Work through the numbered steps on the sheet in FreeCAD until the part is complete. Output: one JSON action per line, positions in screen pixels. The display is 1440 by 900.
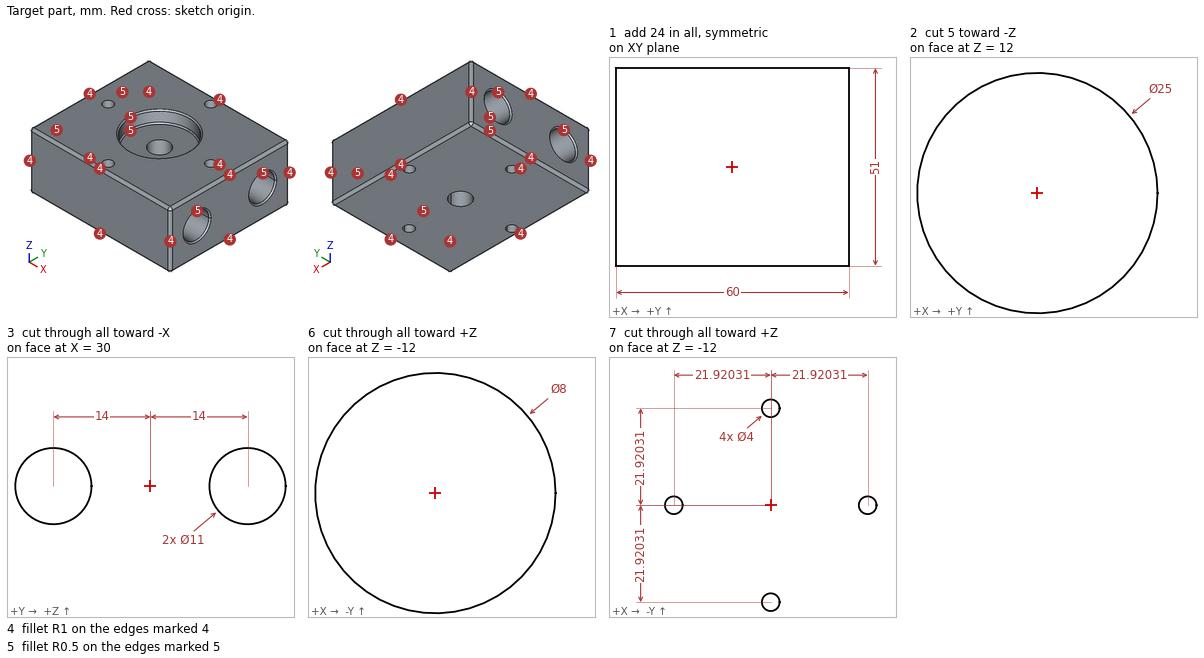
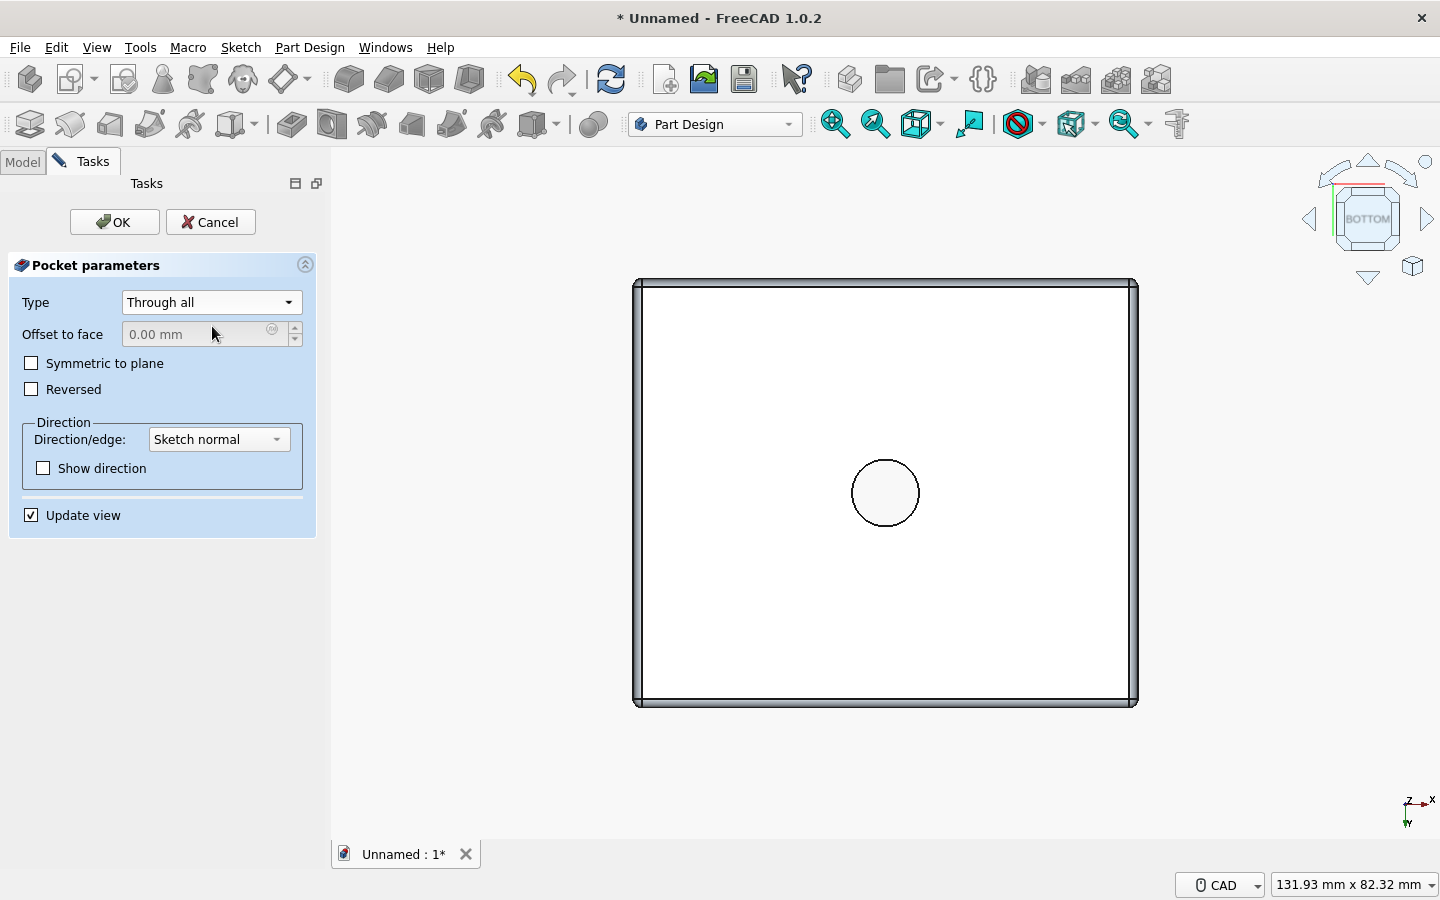
{"action": "left_click", "coordinate": [115, 222]}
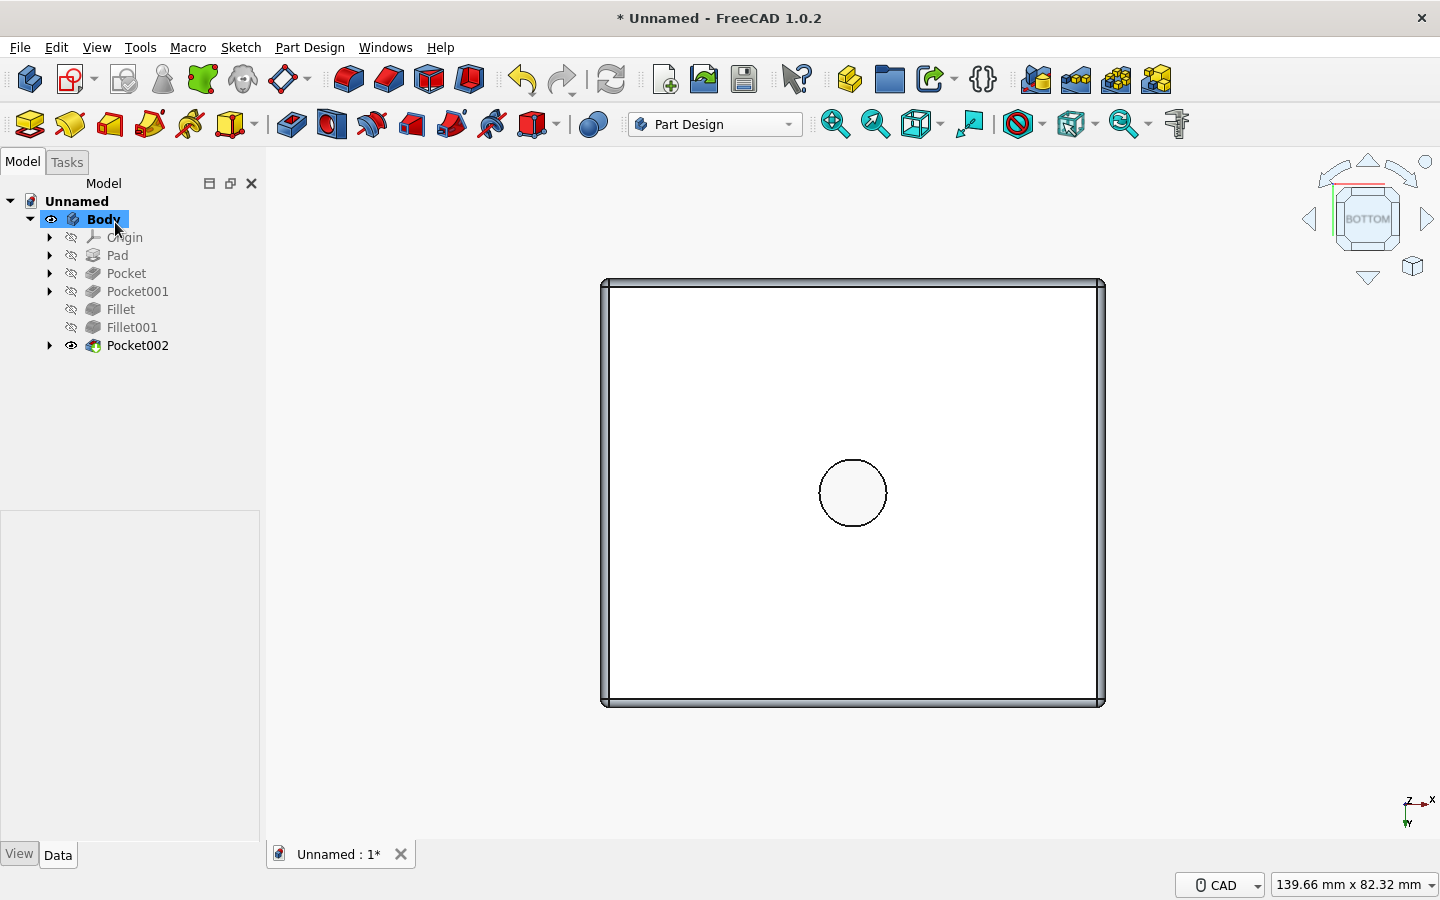
{"action": "left_click", "coordinate": [992, 551]}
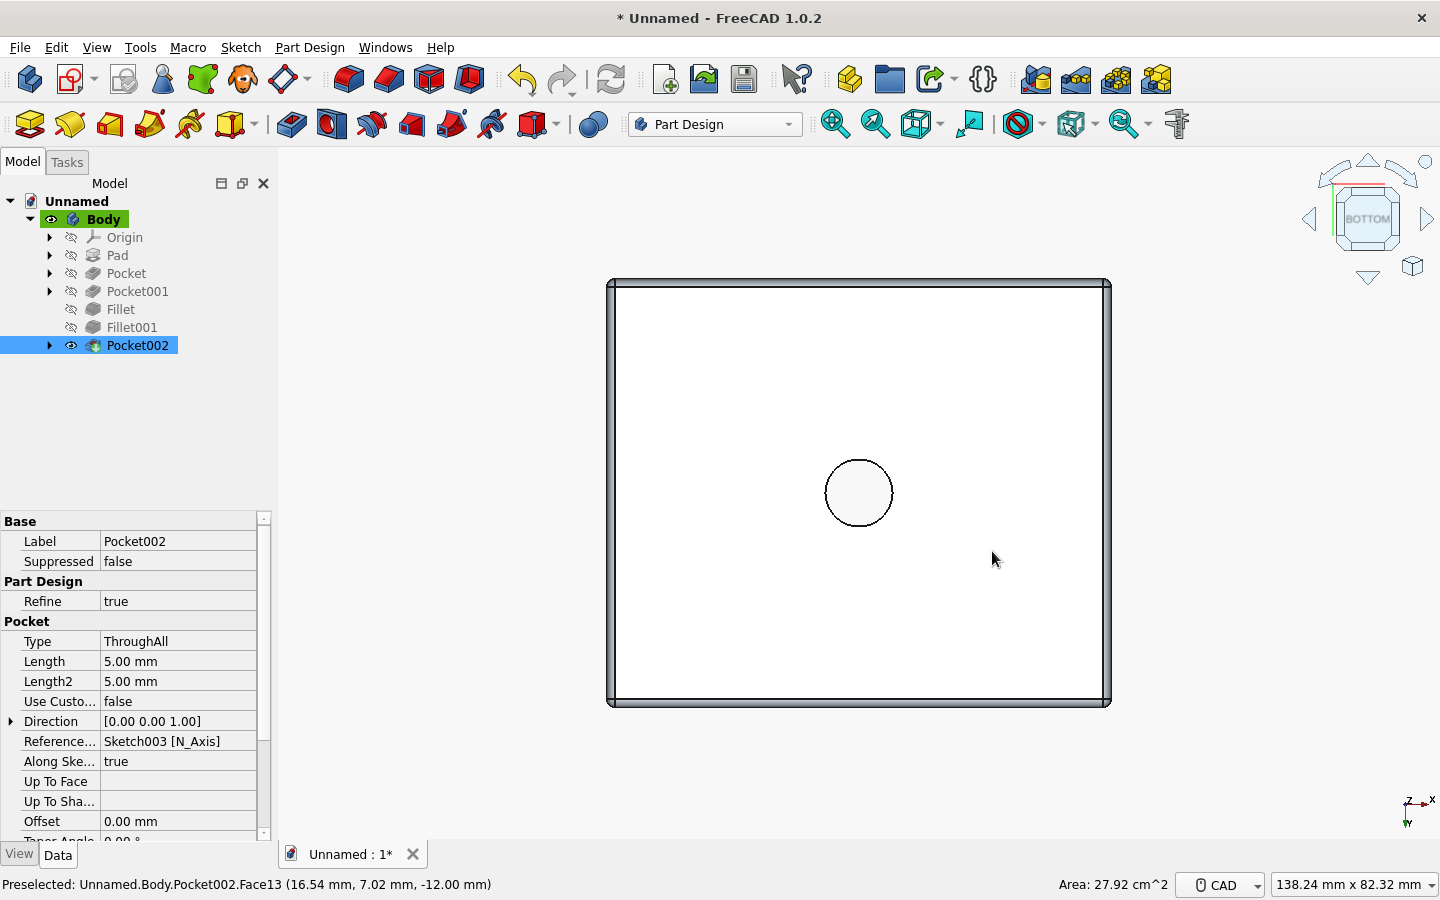
{"action": "left_click", "coordinate": [70, 80]}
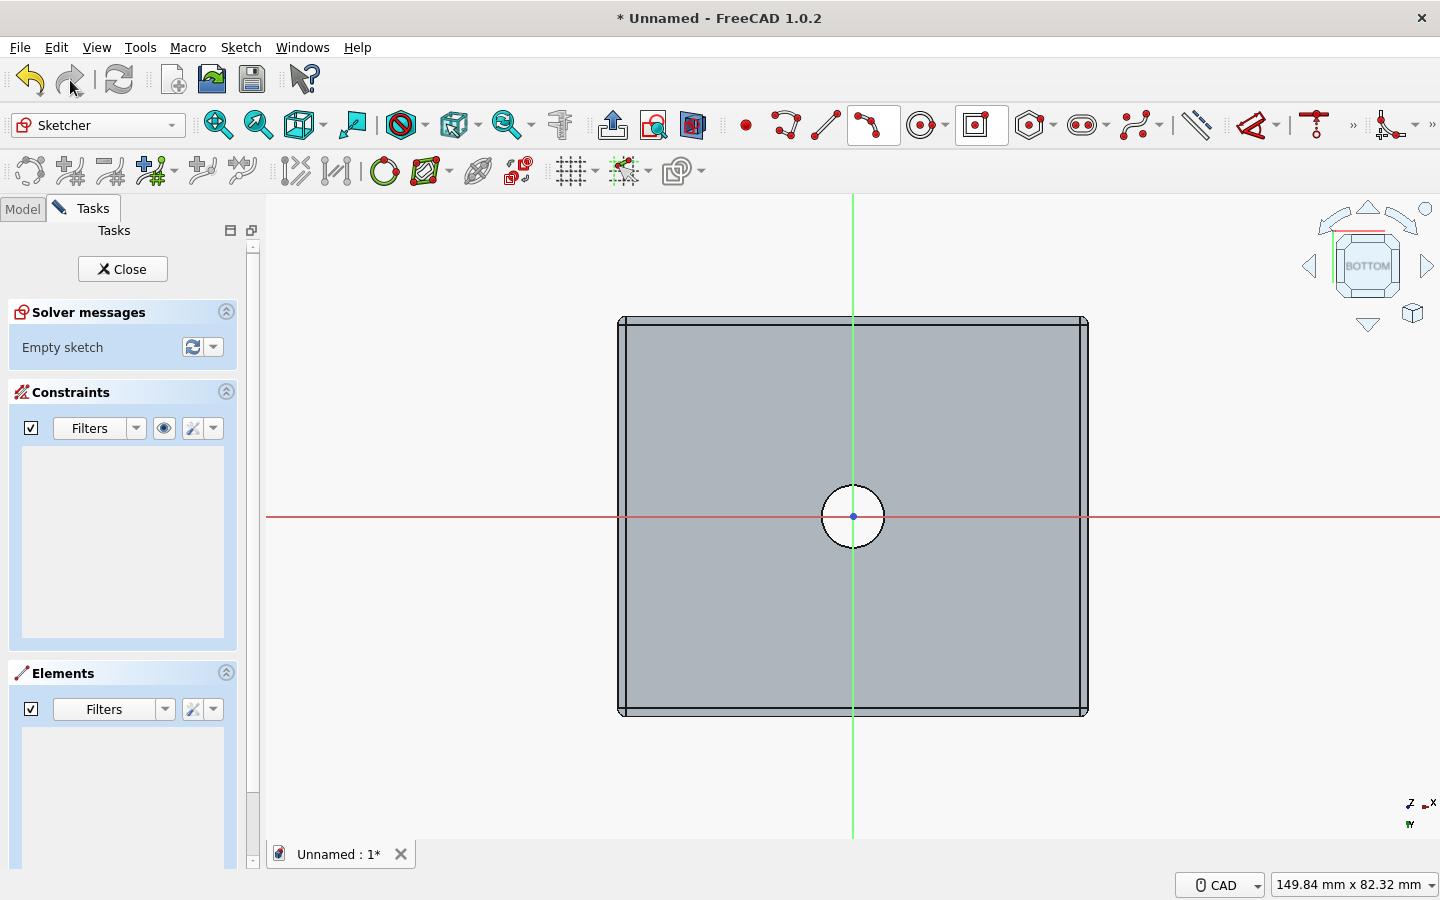
{"action": "left_click", "coordinate": [922, 126]}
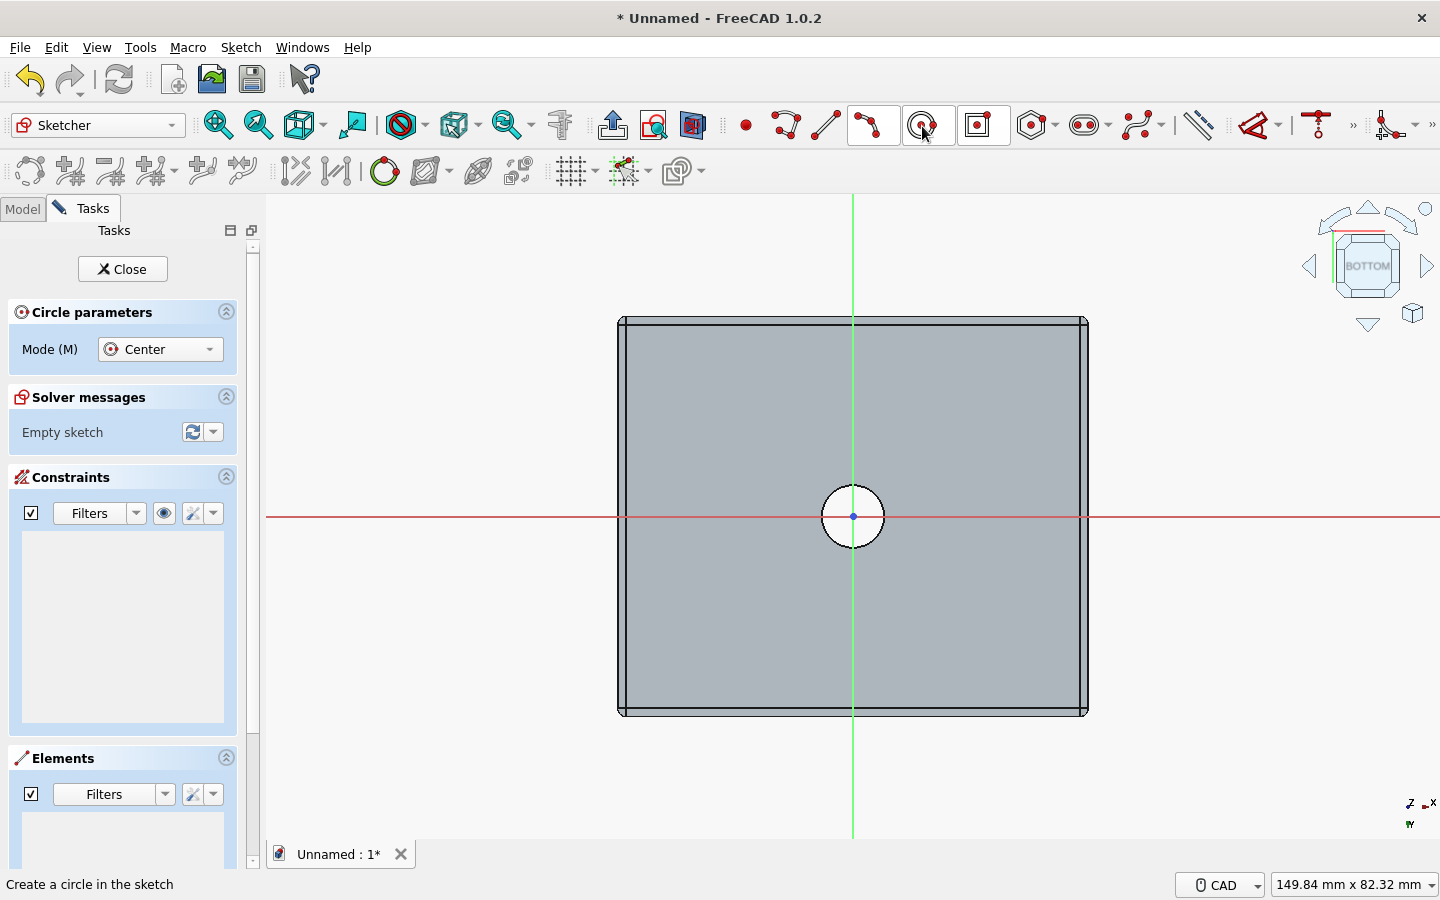
{"action": "scroll", "coordinate": [853, 345], "scroll_direction": "up", "scroll_amount": 2}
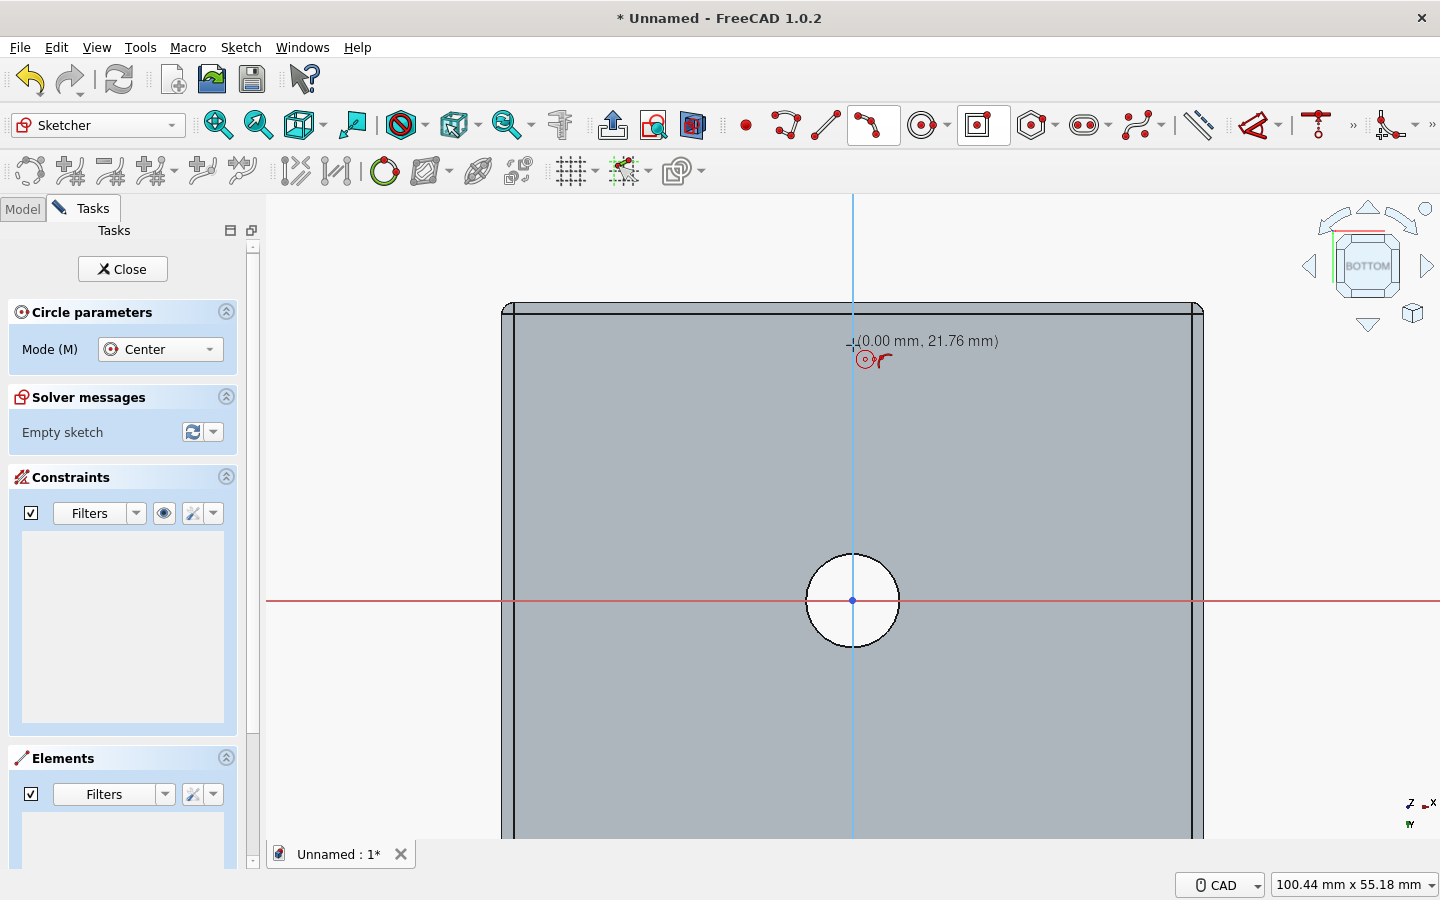
{"action": "left_click", "coordinate": [853, 345]}
{"action": "left_click", "coordinate": [869, 328]}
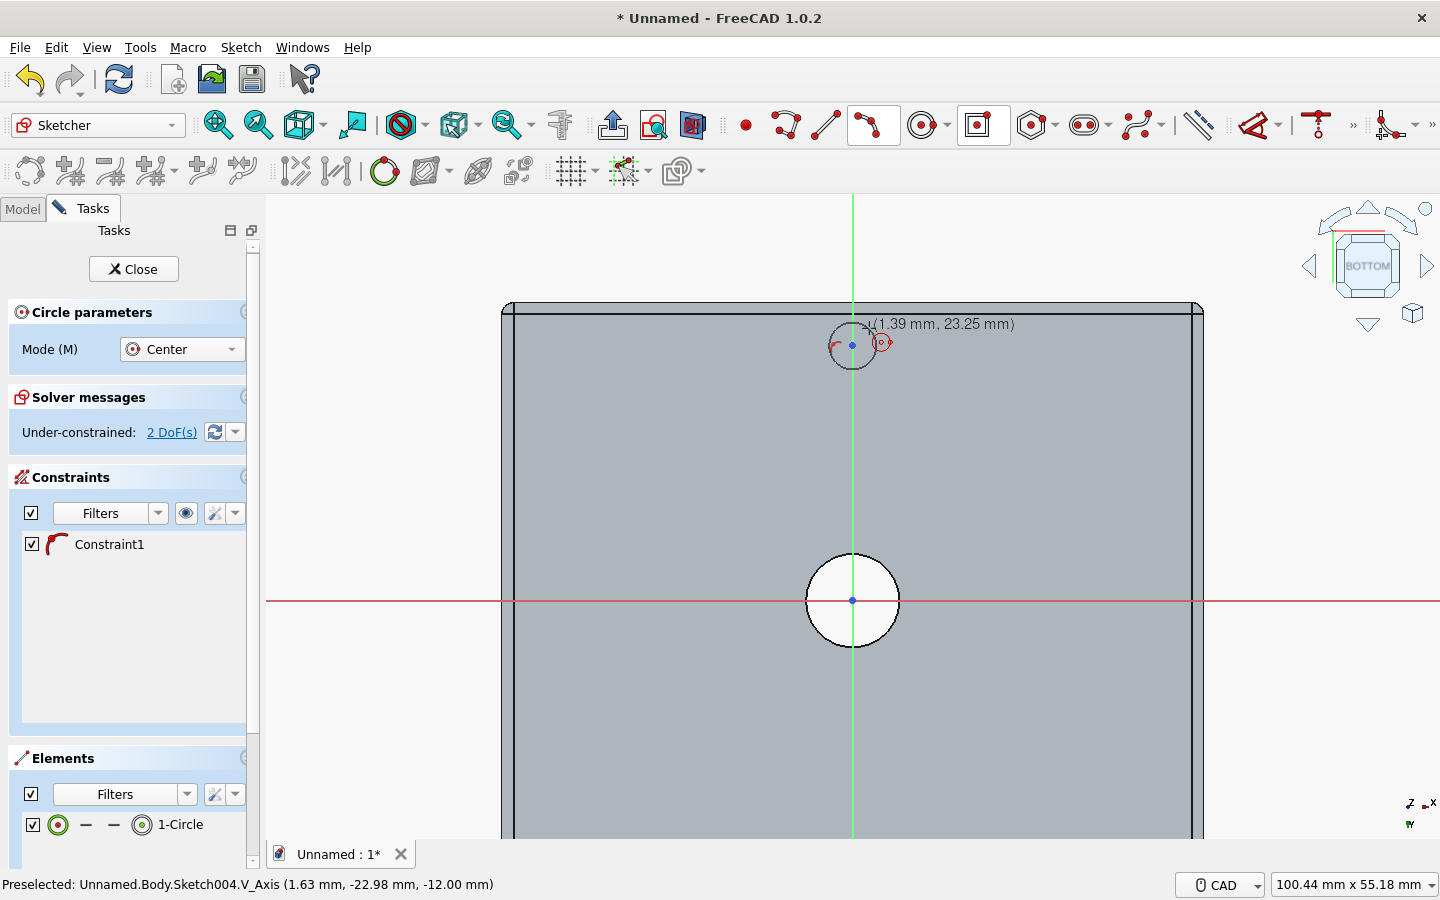
{"action": "left_click", "coordinate": [1109, 601]}
{"action": "left_click", "coordinate": [1125, 584]}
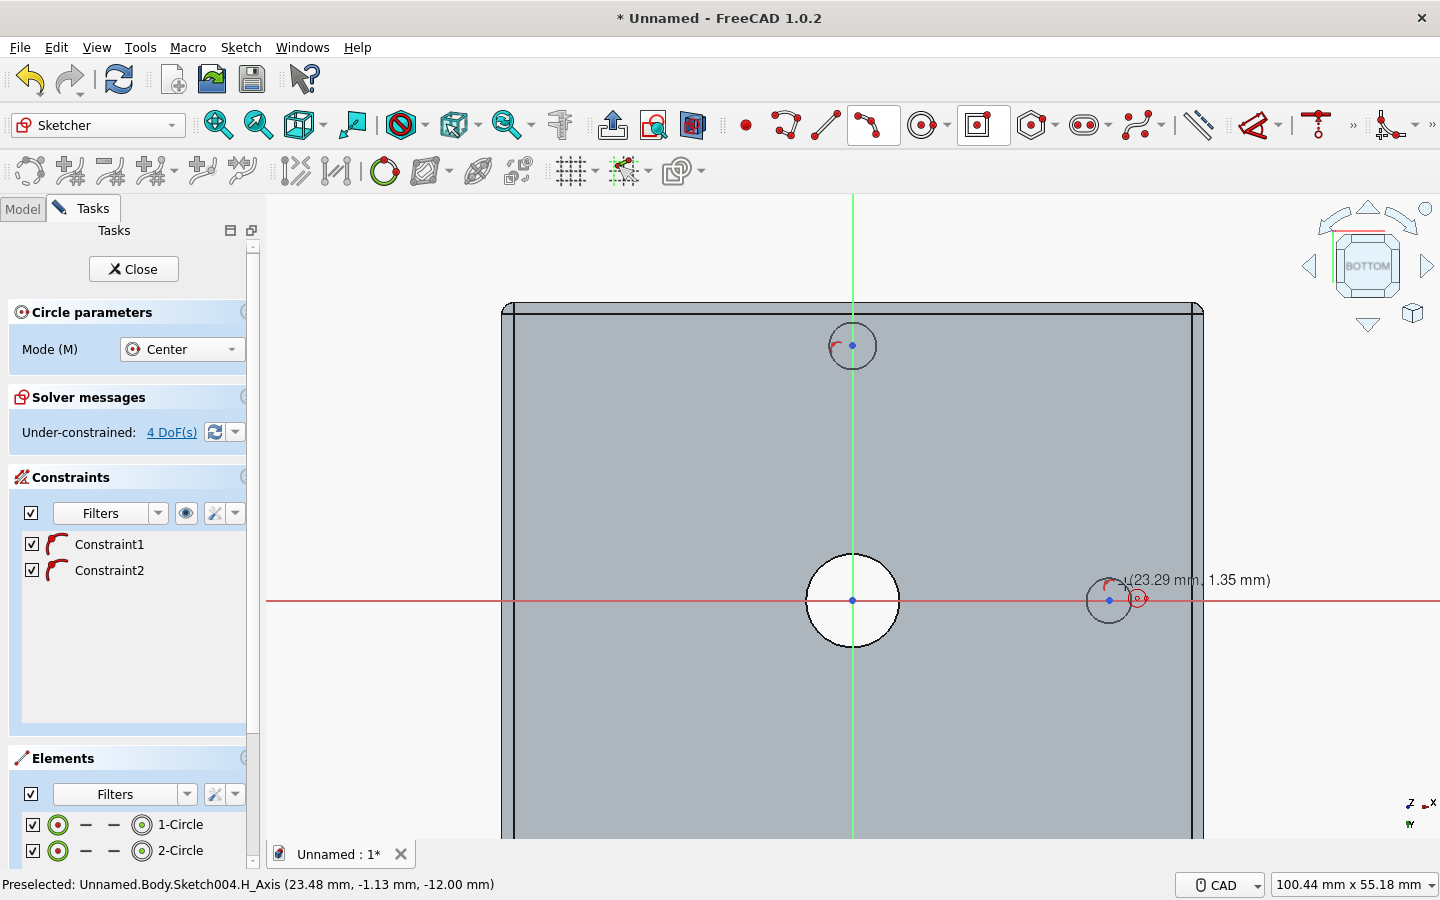
{"action": "scroll", "coordinate": [476, 222], "scroll_direction": "down", "scroll_amount": 1}